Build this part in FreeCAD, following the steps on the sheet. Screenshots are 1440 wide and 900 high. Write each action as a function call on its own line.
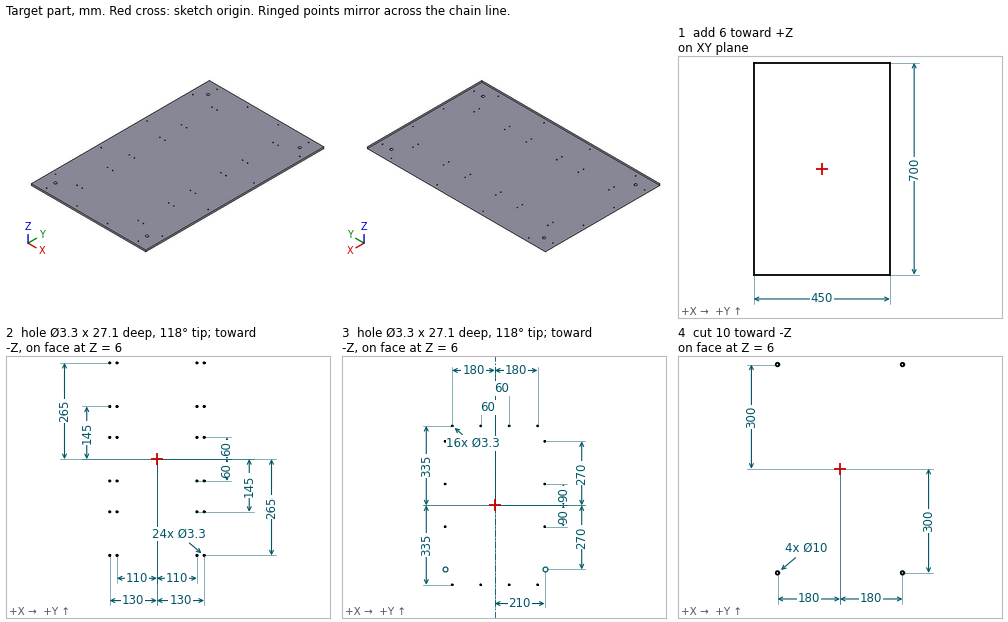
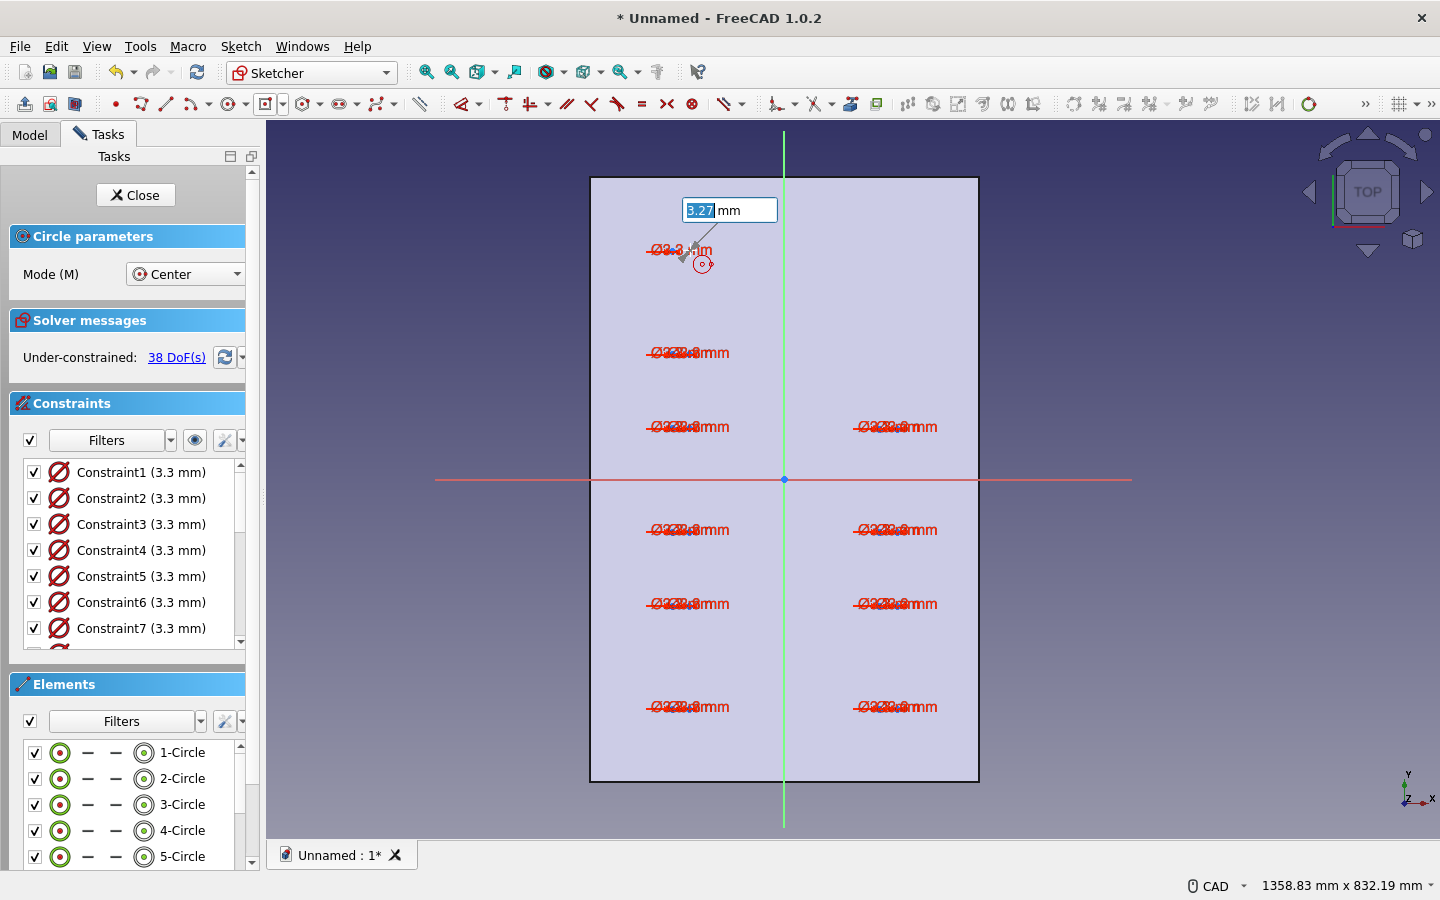
text(3.3)
key(Return)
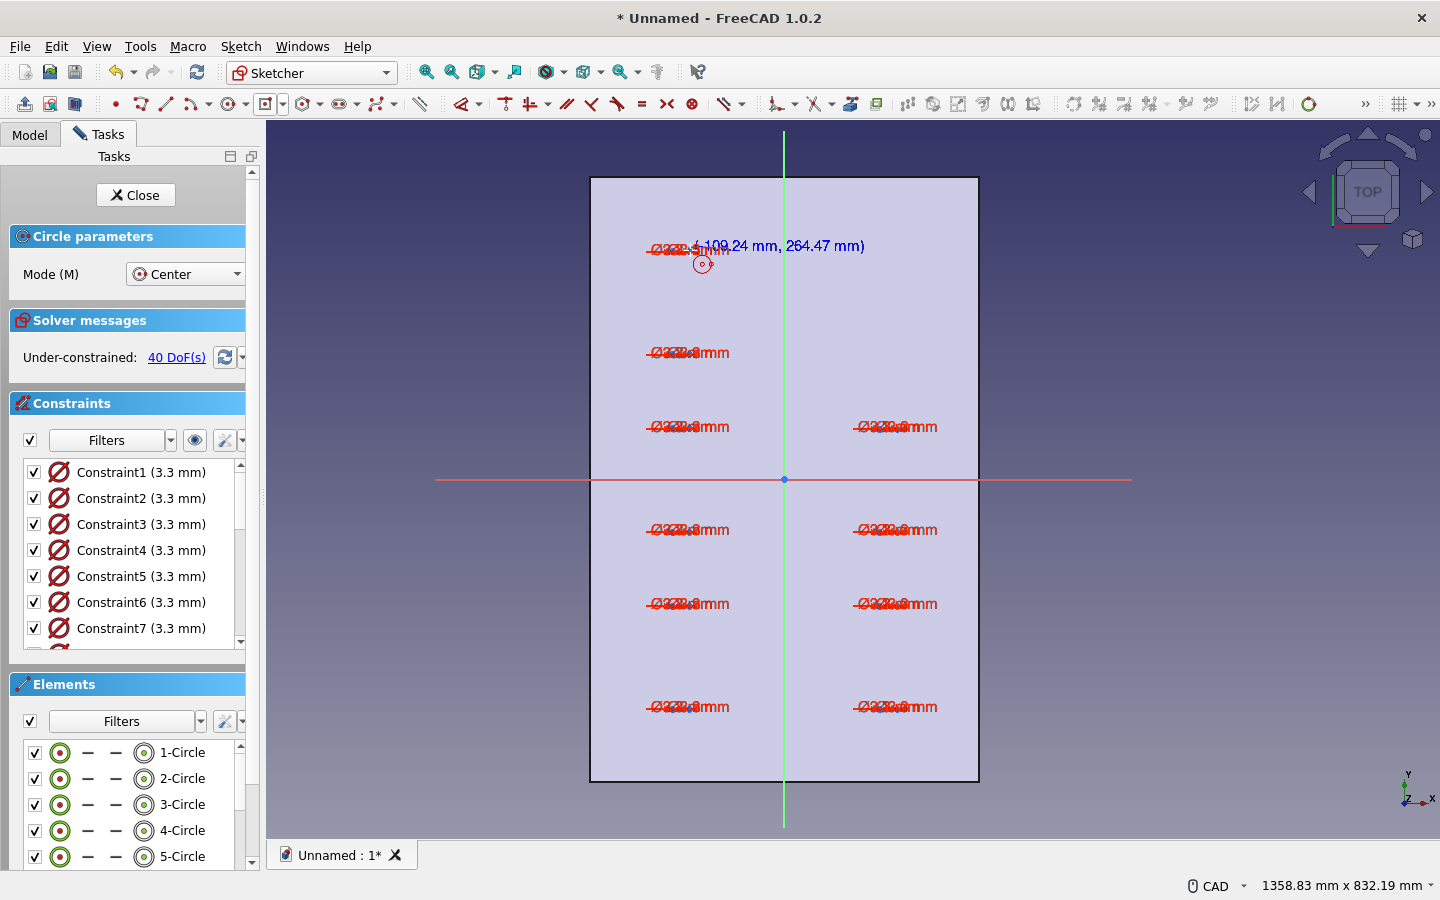
scroll(879, 354, up, 14)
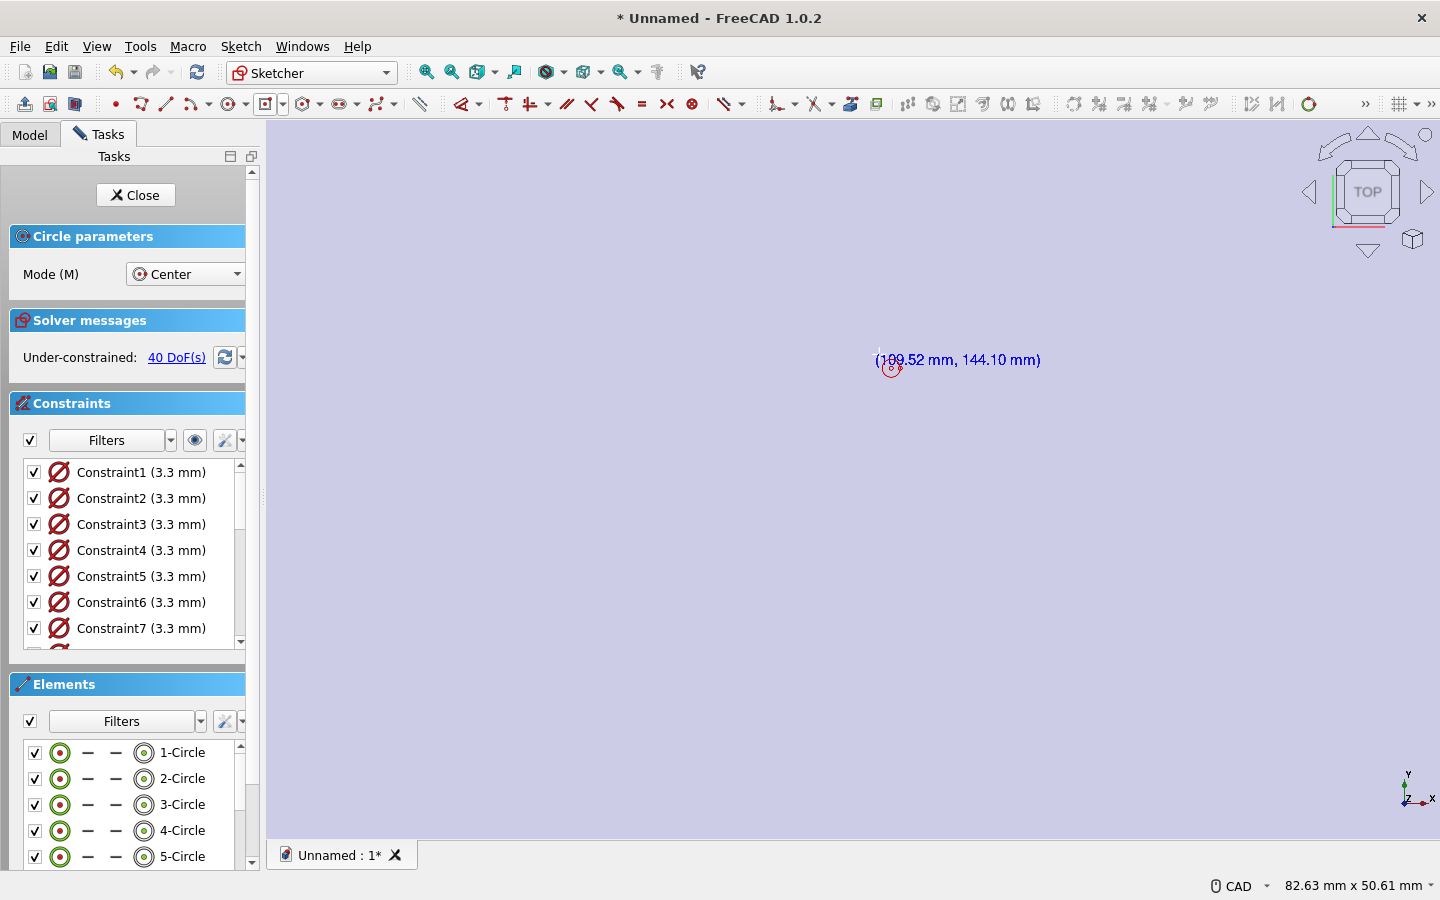
scroll(880, 354, down, 14)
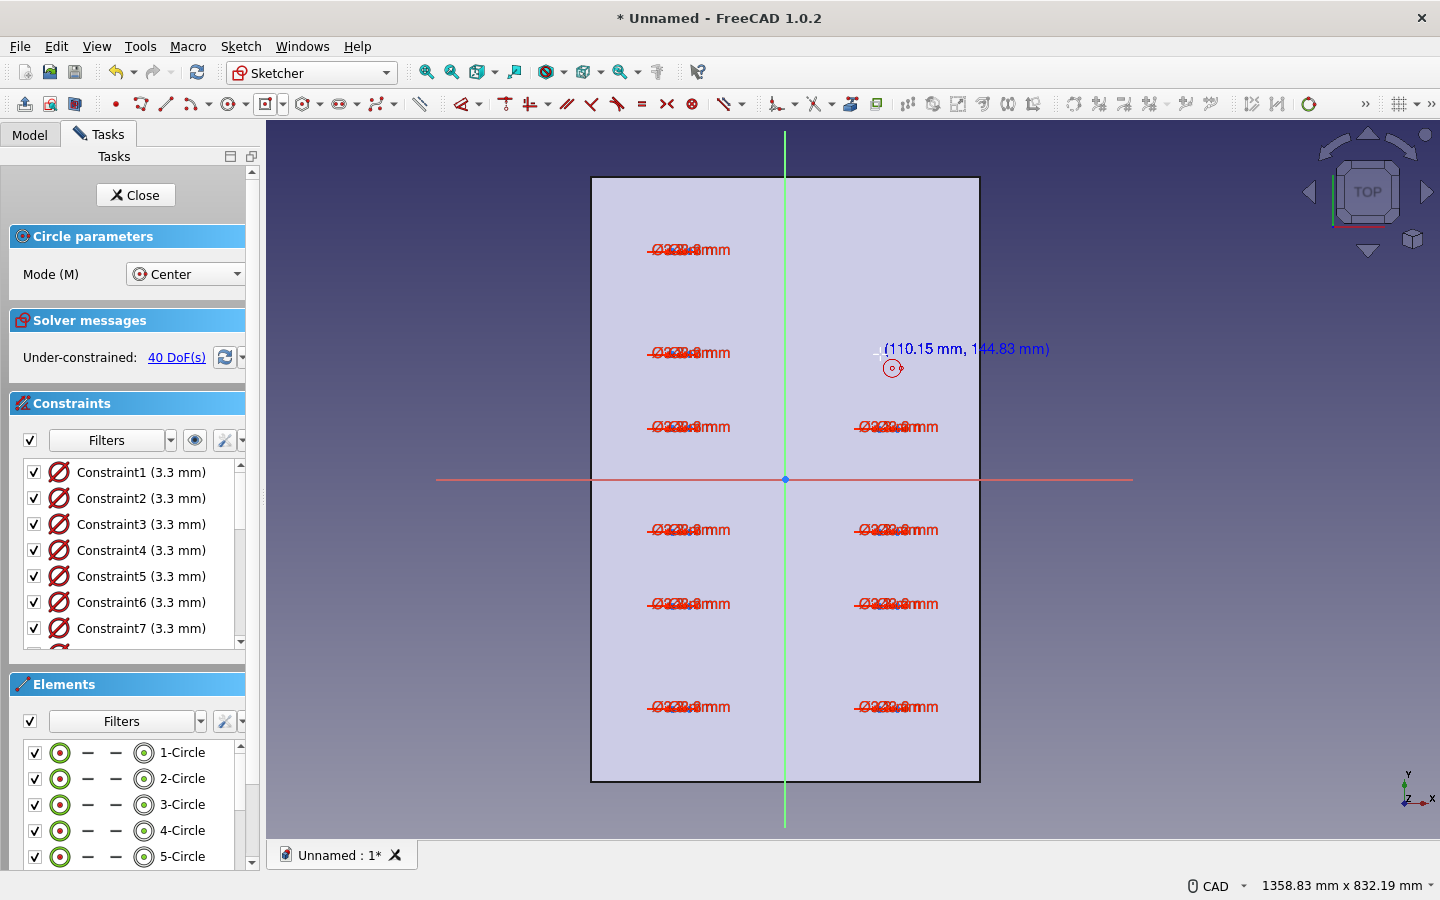
click(880, 354)
move(881, 353)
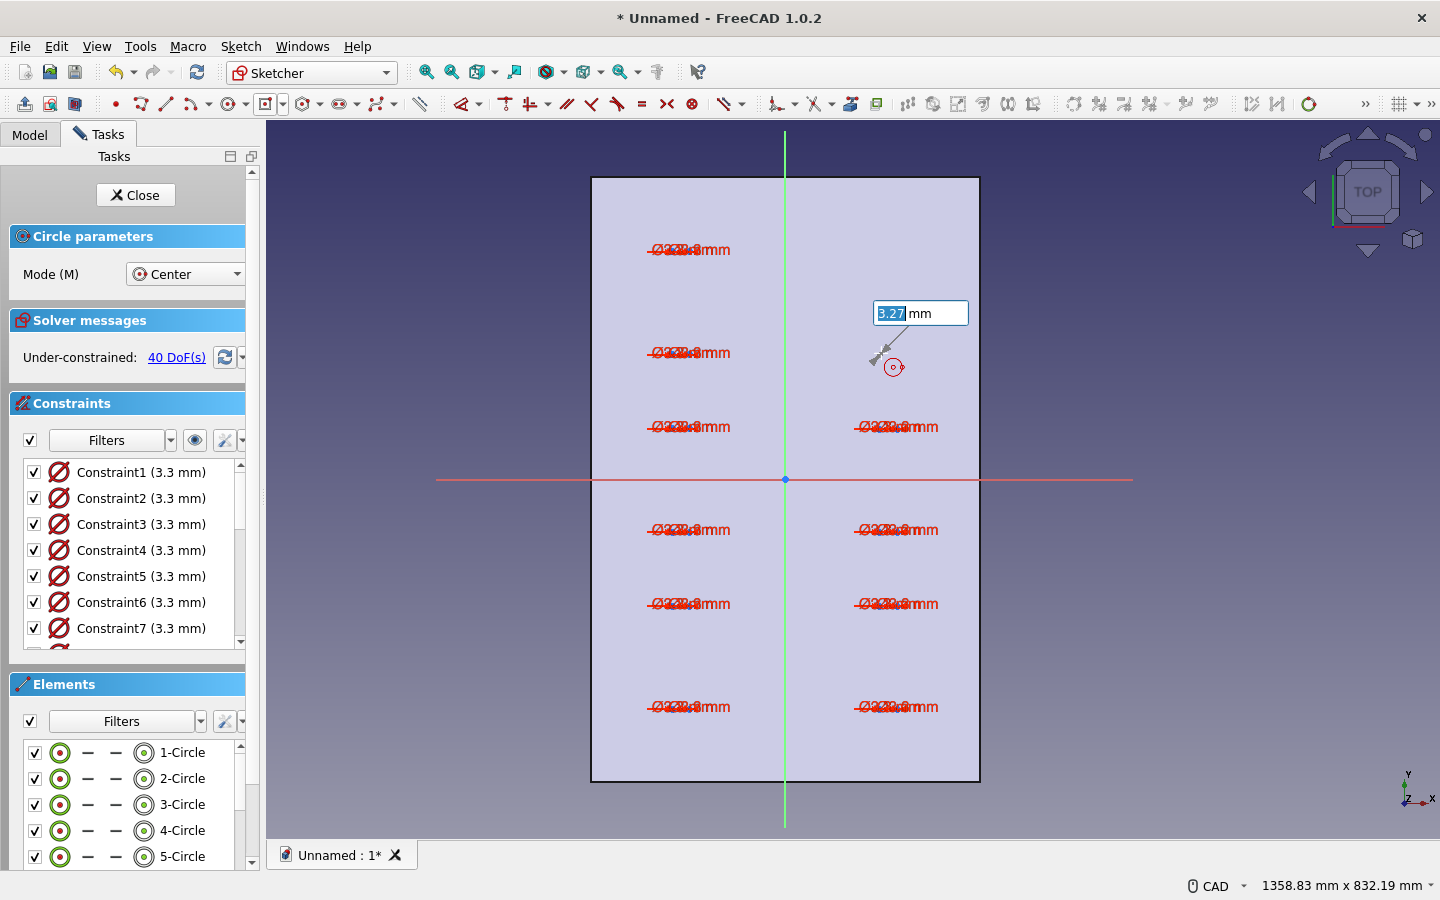
text(3.3)
key(Return)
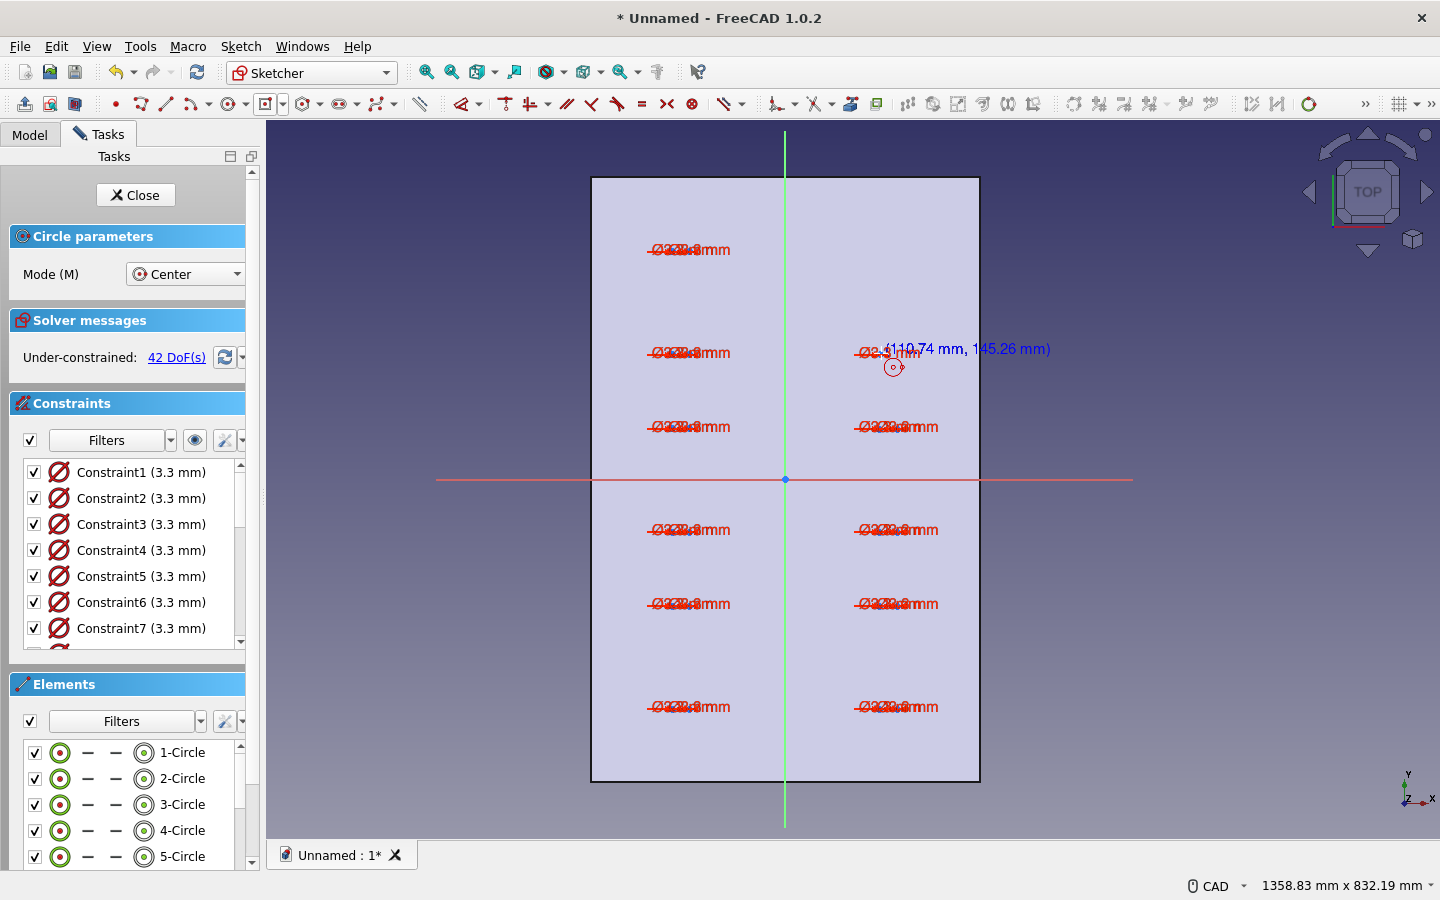
scroll(898, 354, up, 14)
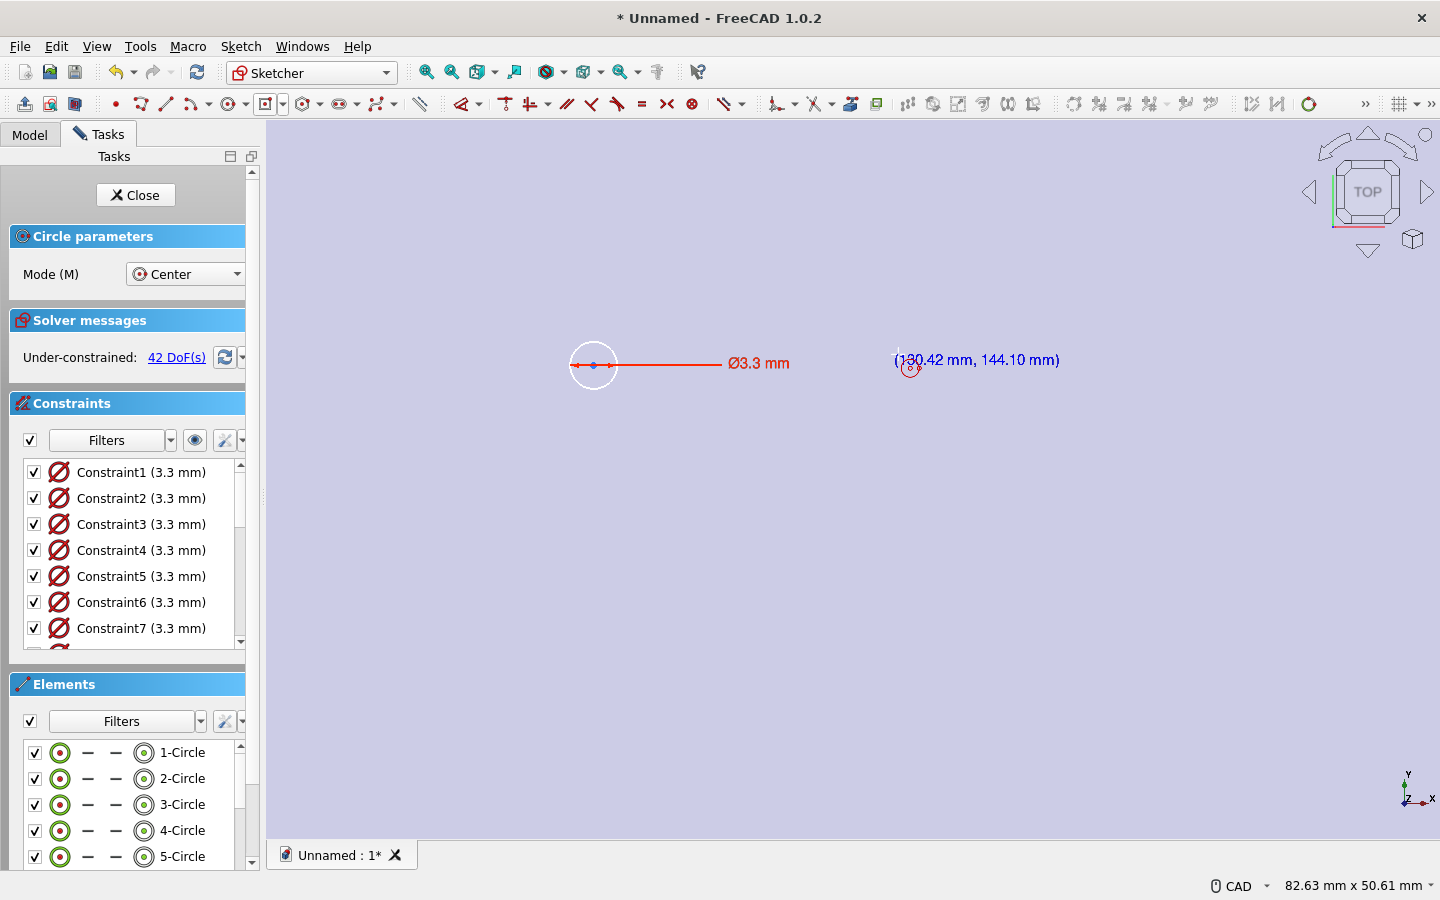
scroll(898, 354, down, 14)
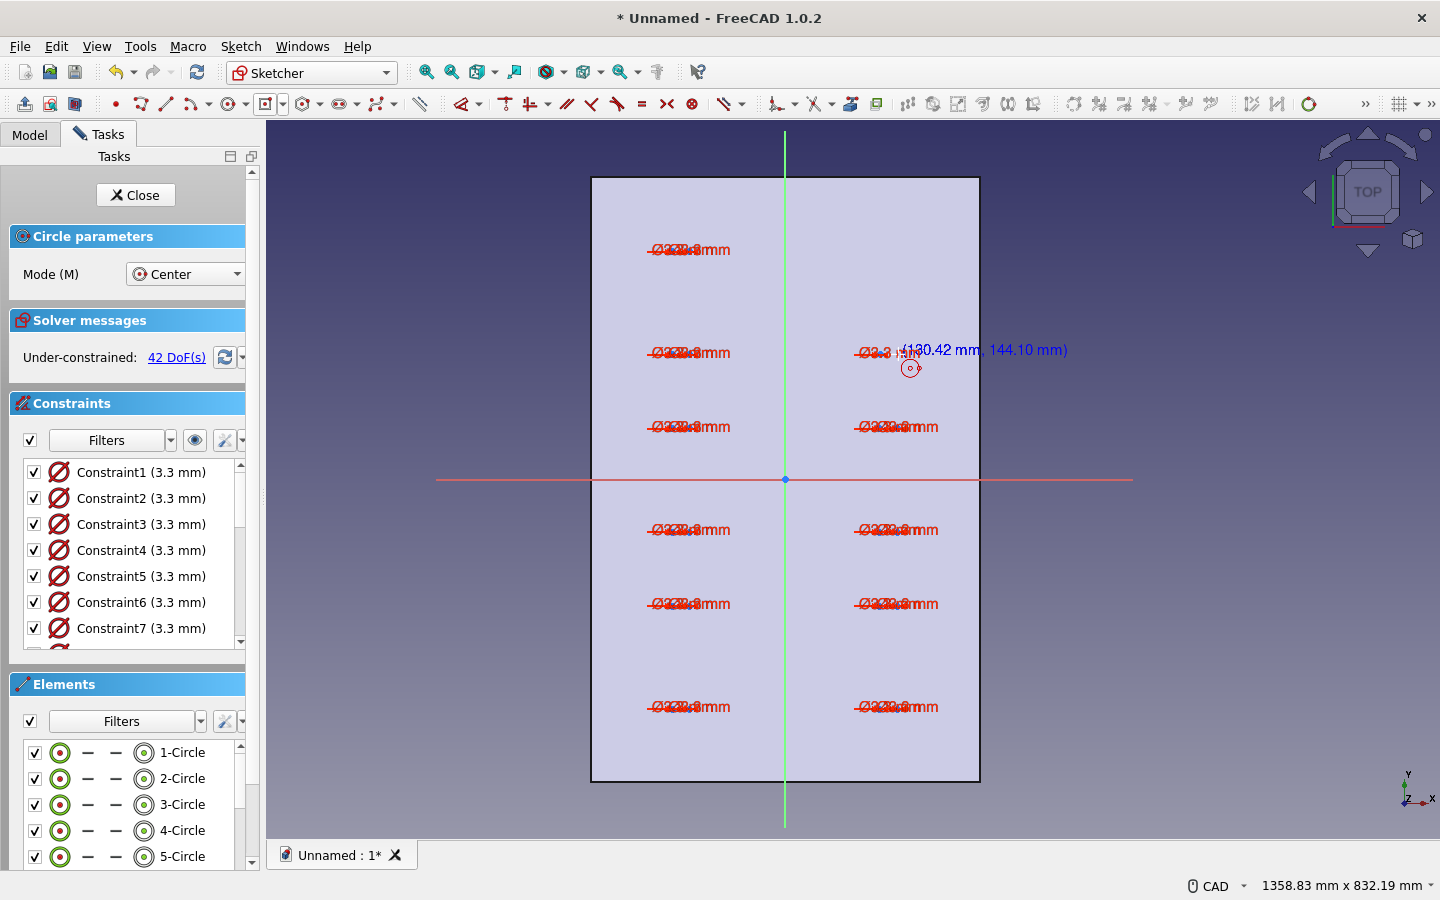
click(898, 354)
move(899, 353)